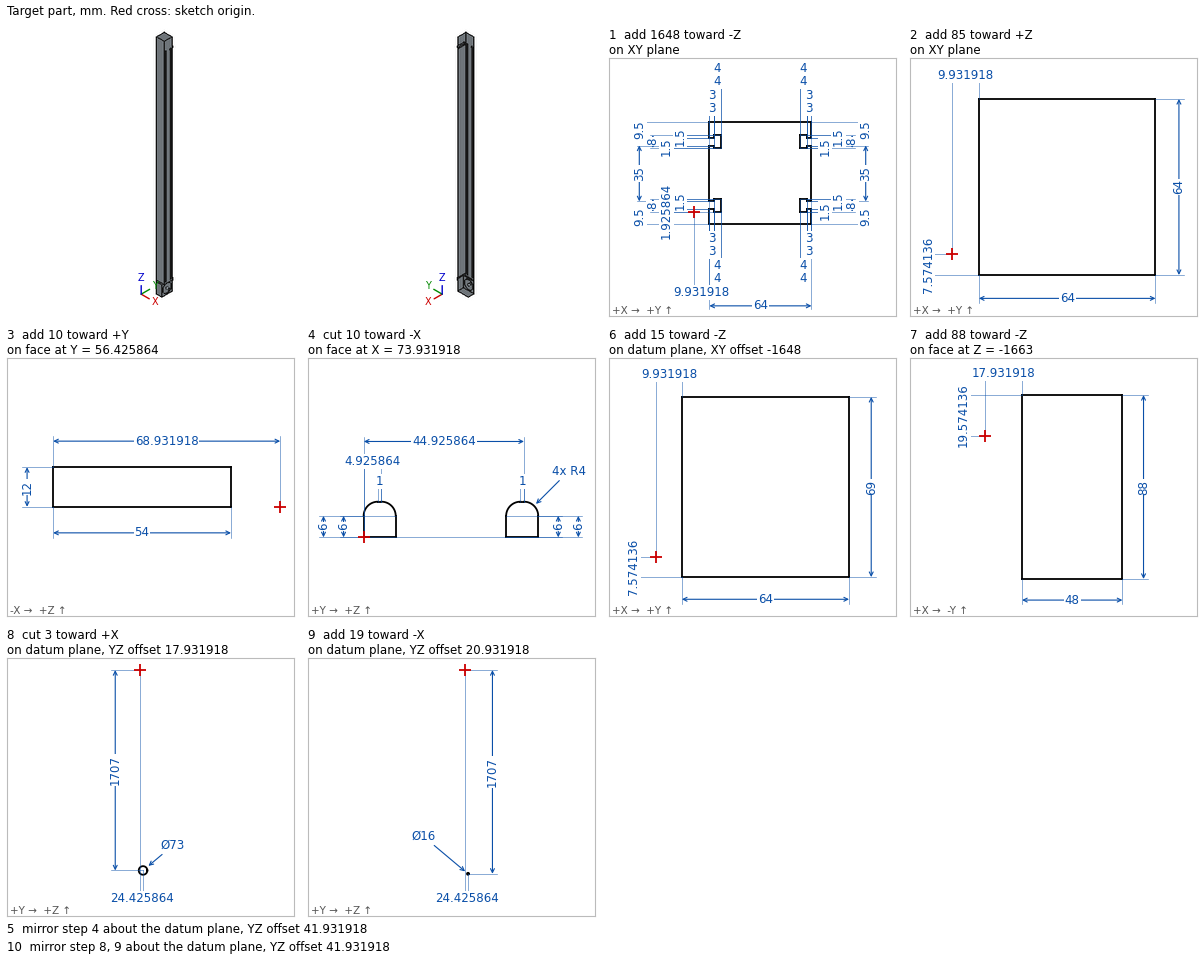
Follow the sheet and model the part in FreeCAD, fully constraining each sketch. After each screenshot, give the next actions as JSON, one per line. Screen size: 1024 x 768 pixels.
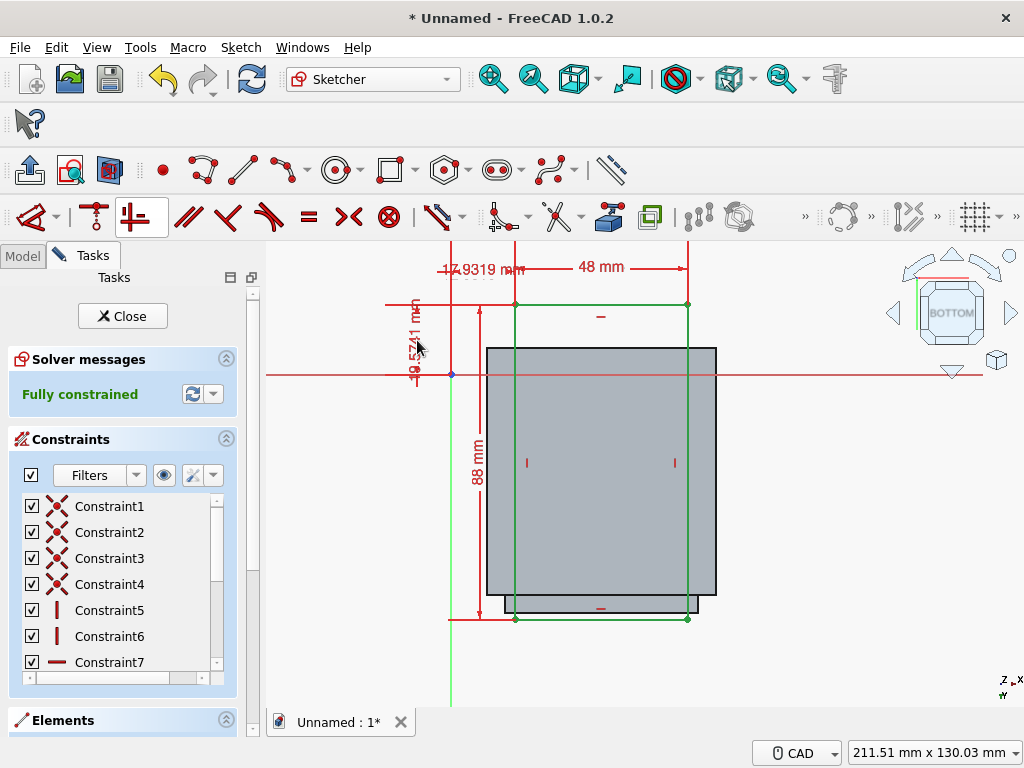
{"action": "left_click", "coordinate": [123, 316]}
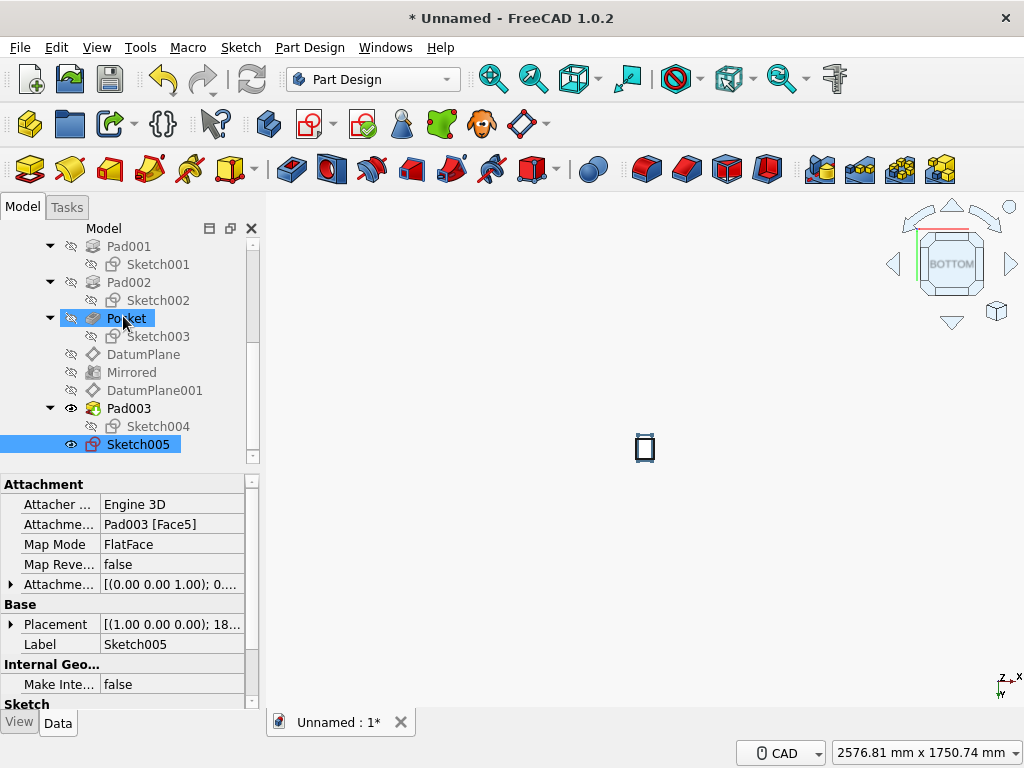
{"action": "left_click", "coordinate": [30, 170]}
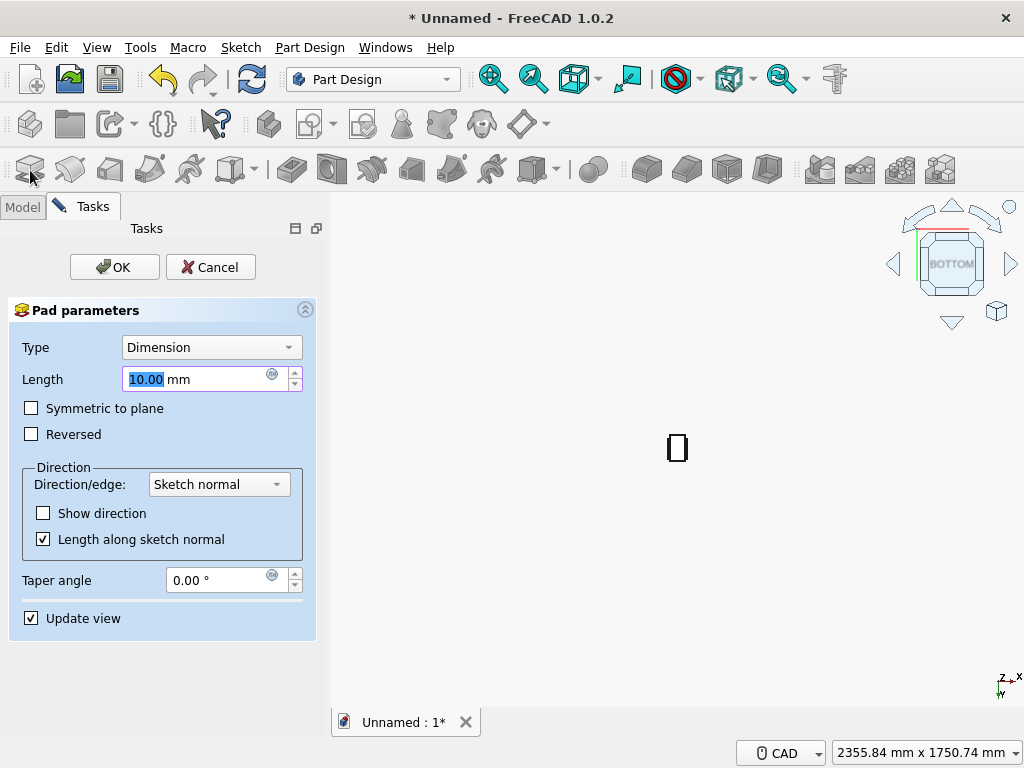
{"action": "type", "text": "88"}
{"action": "key", "text": "Tab"}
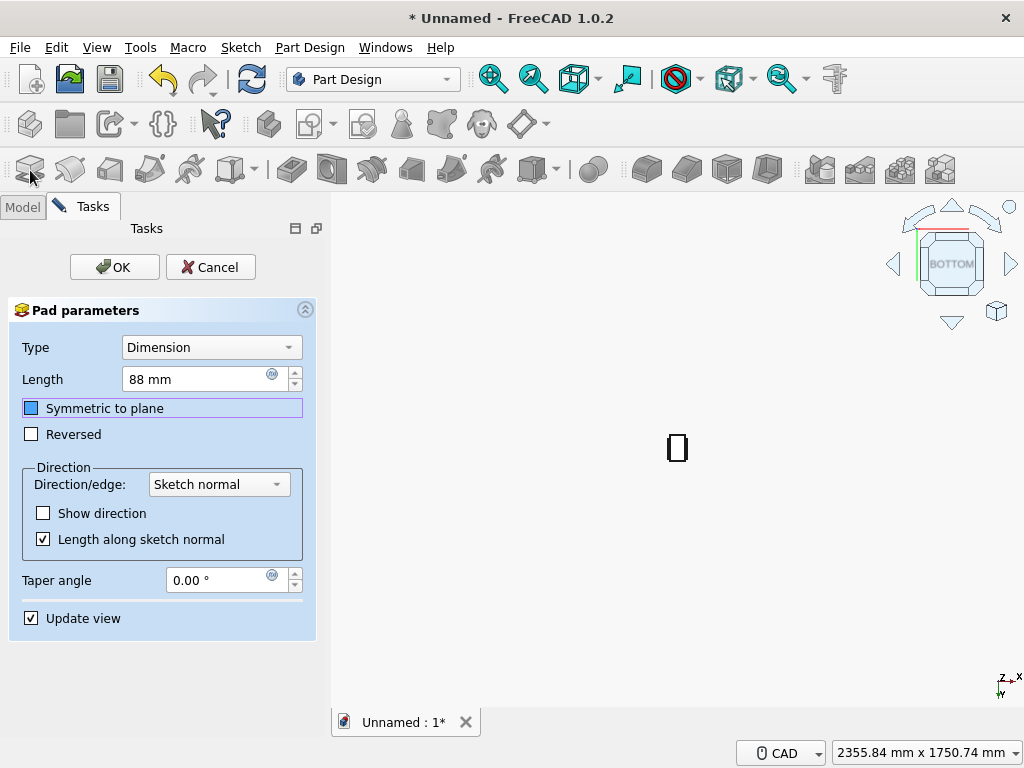
{"action": "left_click", "coordinate": [115, 267]}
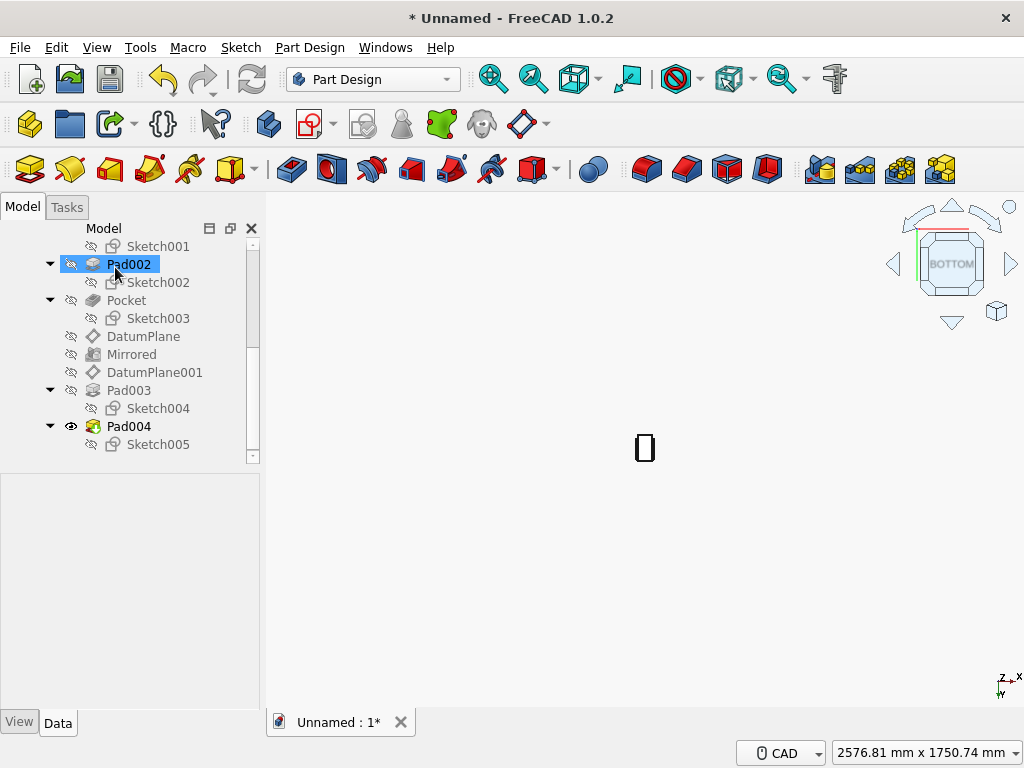
{"action": "left_click", "coordinate": [494, 80]}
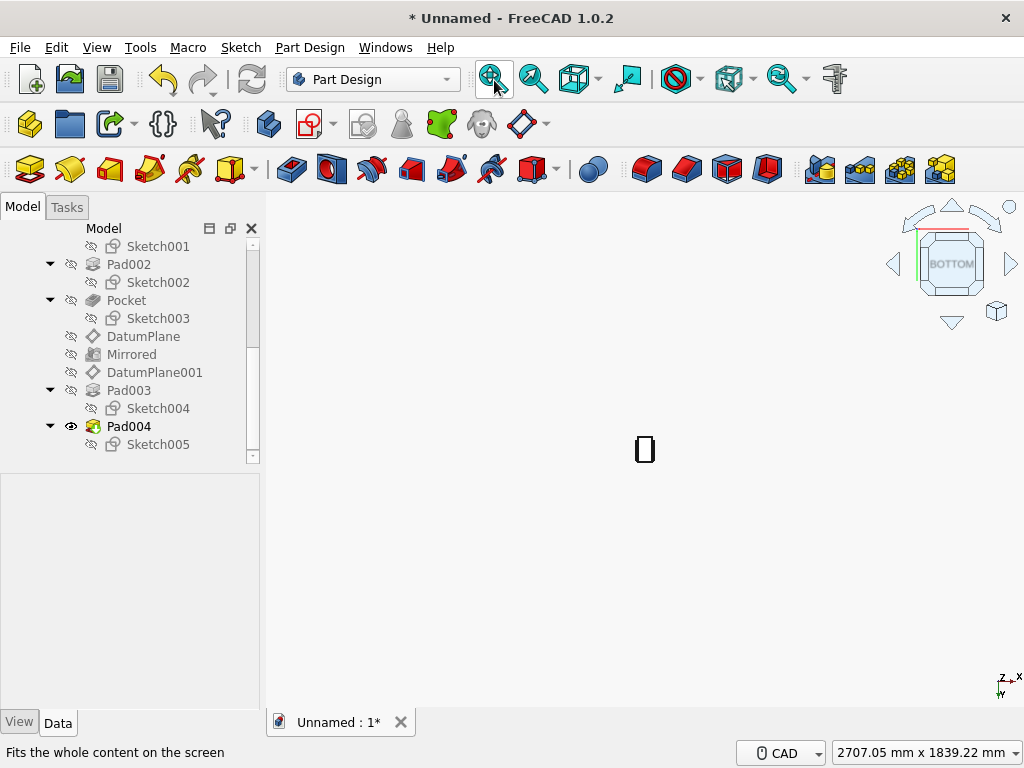
{"action": "key", "text": "6"}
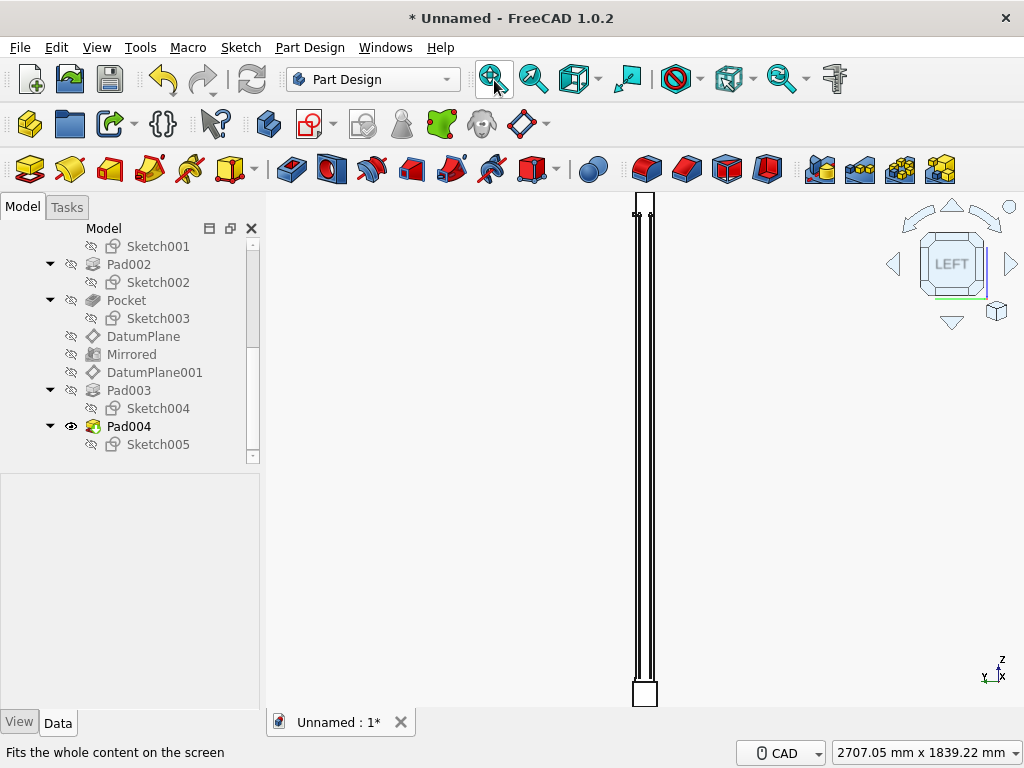
{"action": "left_click", "coordinate": [494, 80]}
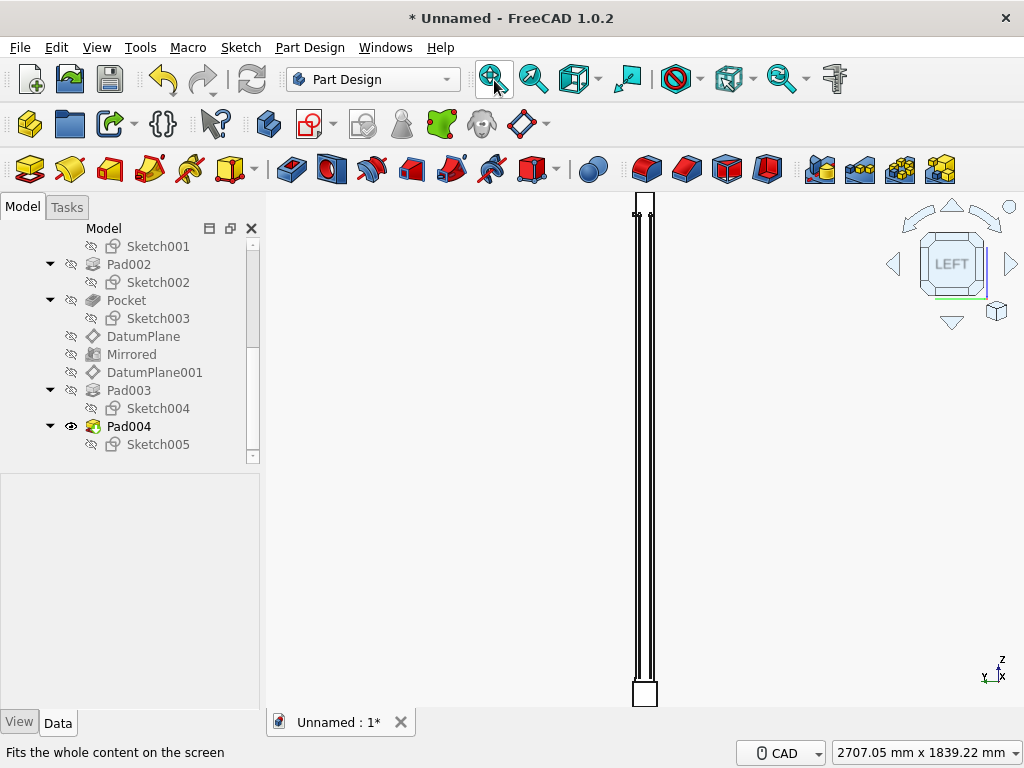
{"action": "key", "text": "2"}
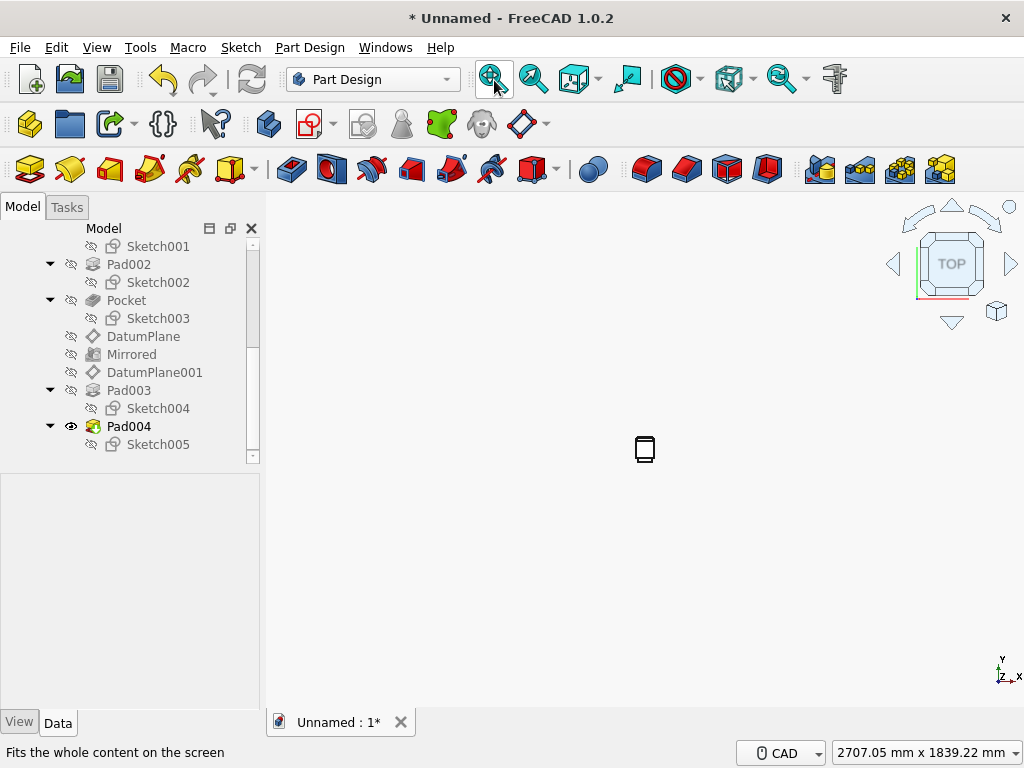
{"action": "left_click", "coordinate": [494, 80]}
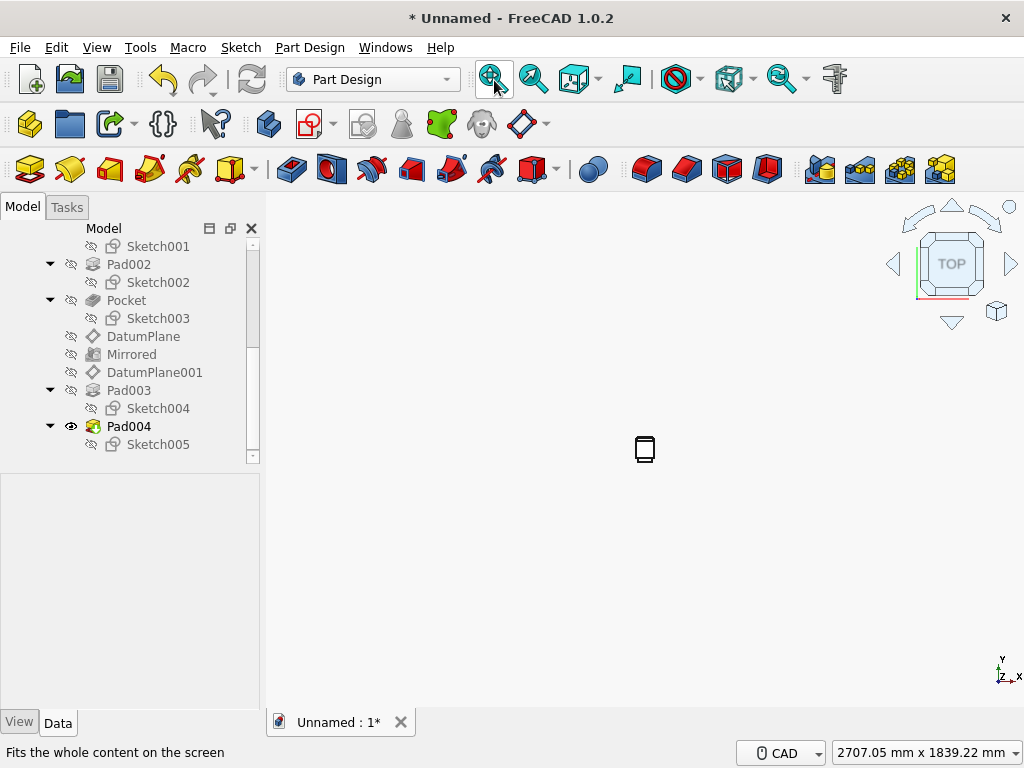
{"action": "key", "text": "1"}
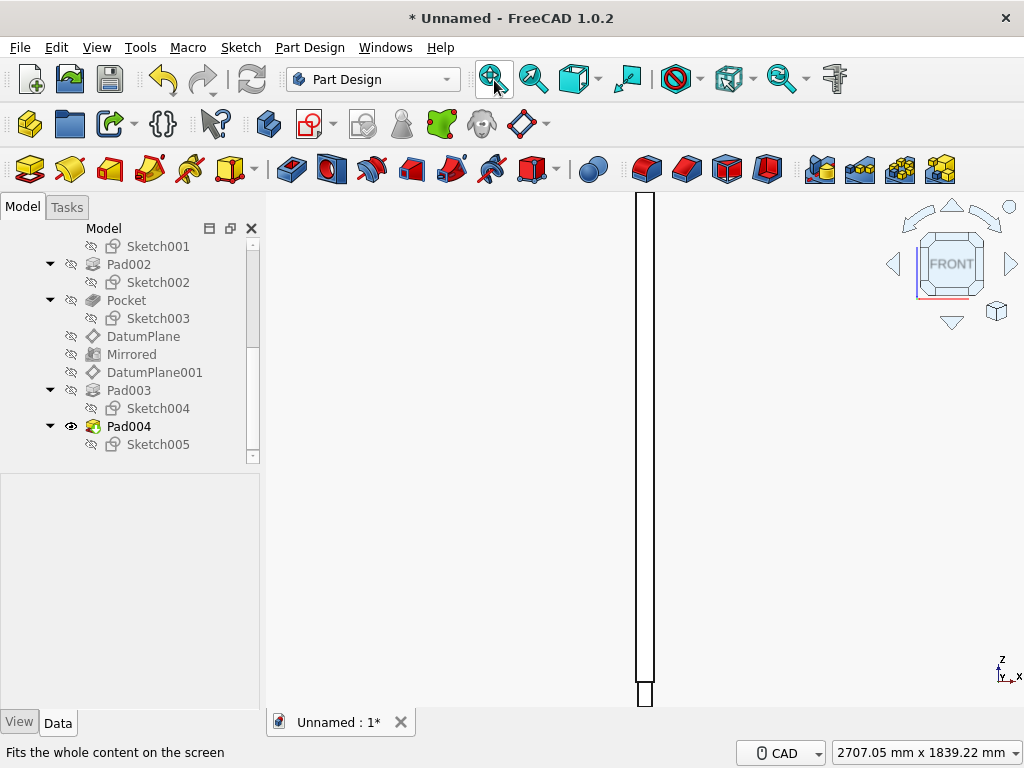
{"action": "left_click", "coordinate": [494, 80]}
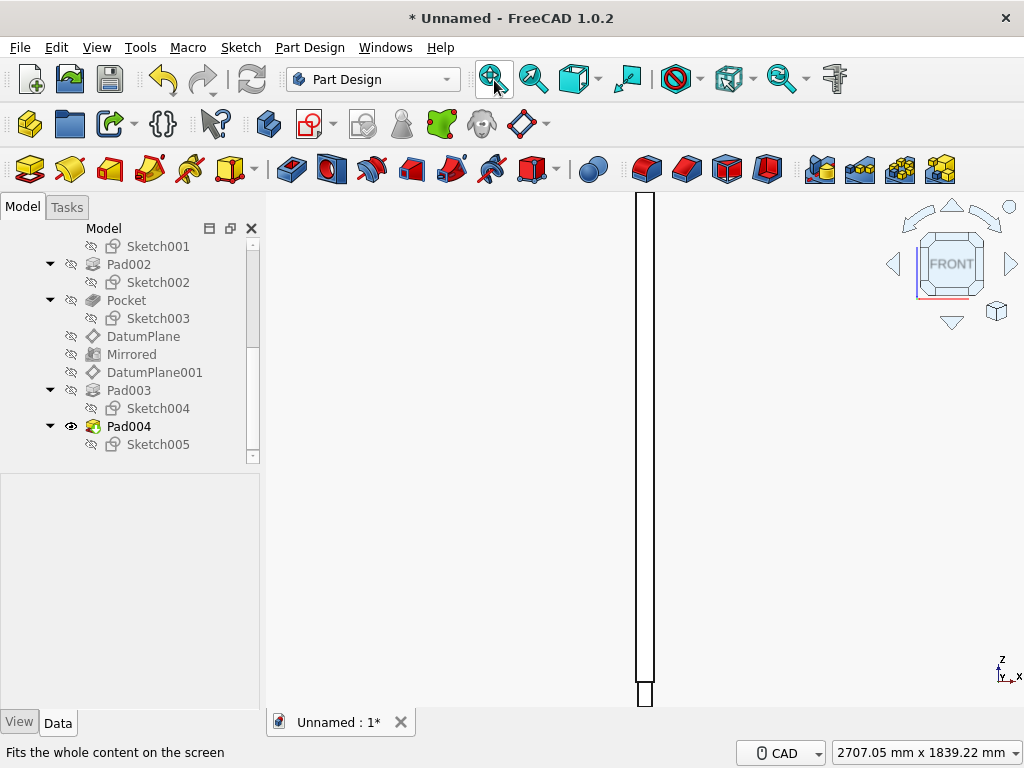
{"action": "scroll", "coordinate": [160, 350], "scroll_direction": "down", "scroll_amount": 3}